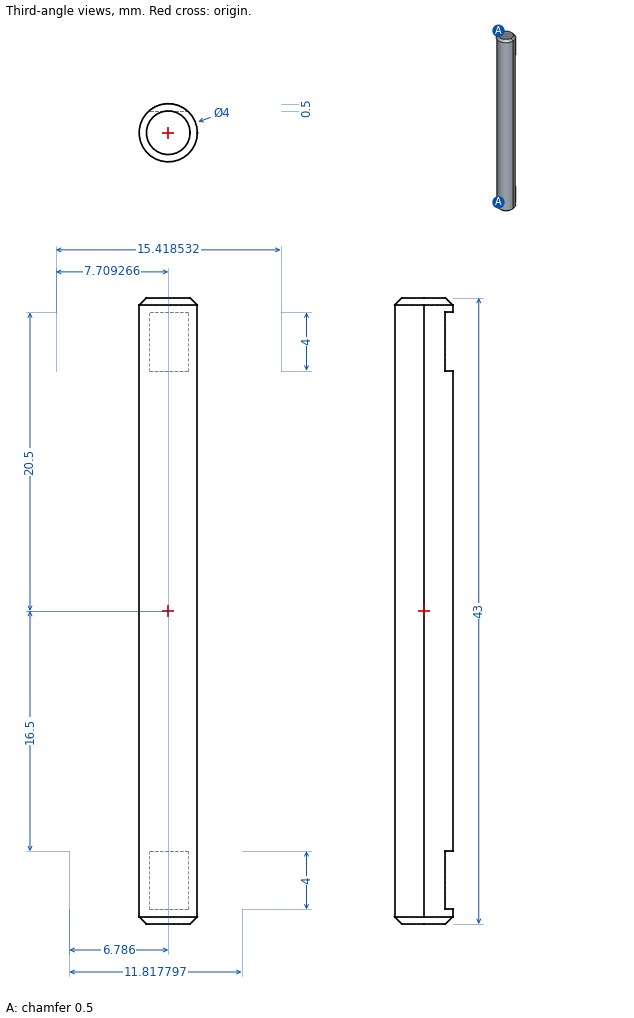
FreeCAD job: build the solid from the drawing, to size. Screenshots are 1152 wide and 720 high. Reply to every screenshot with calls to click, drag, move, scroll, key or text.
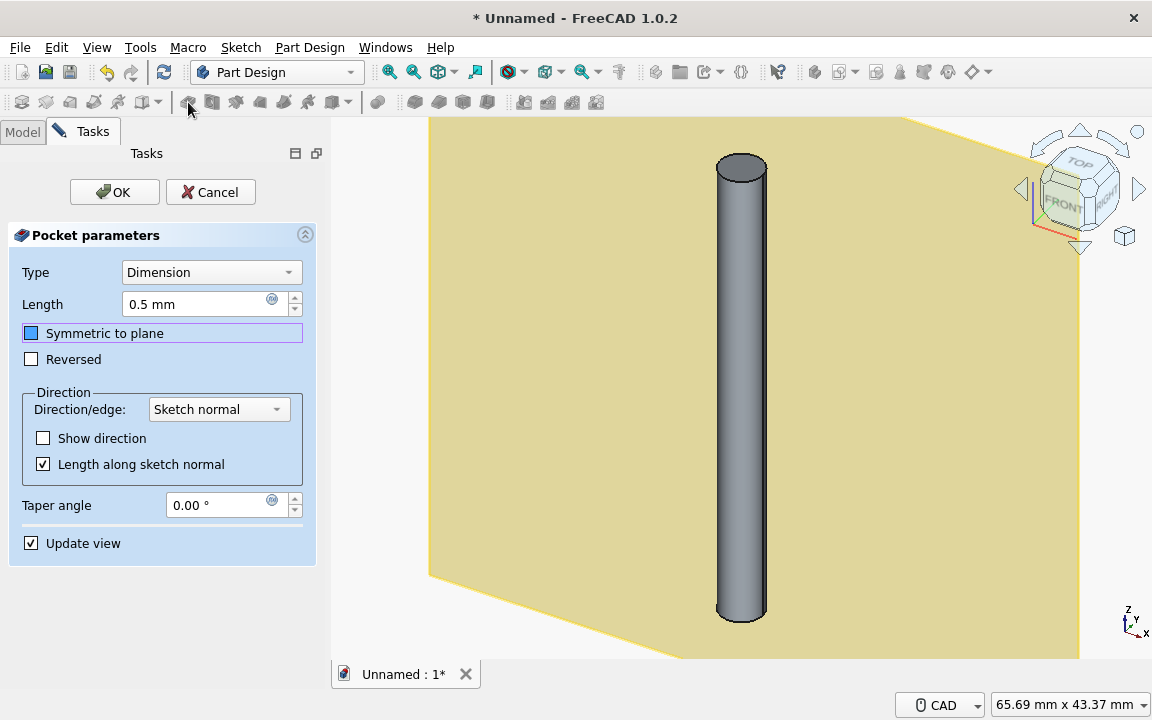
click(30, 359)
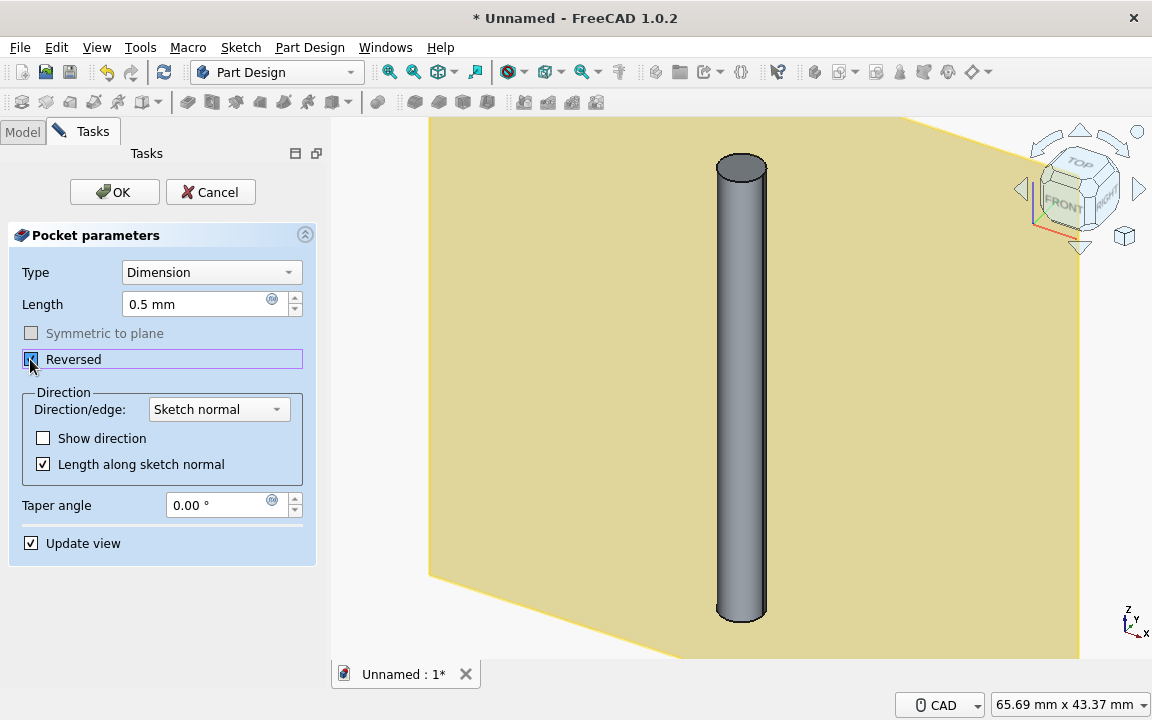
click(115, 192)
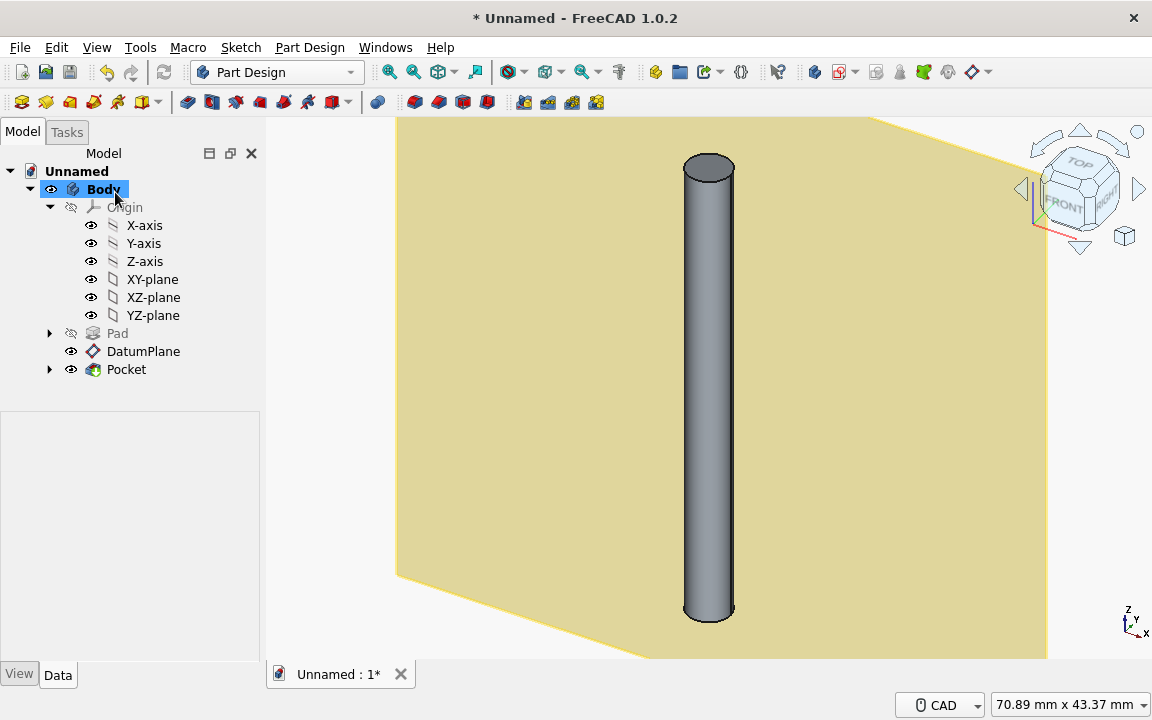
click(116, 351)
key(space)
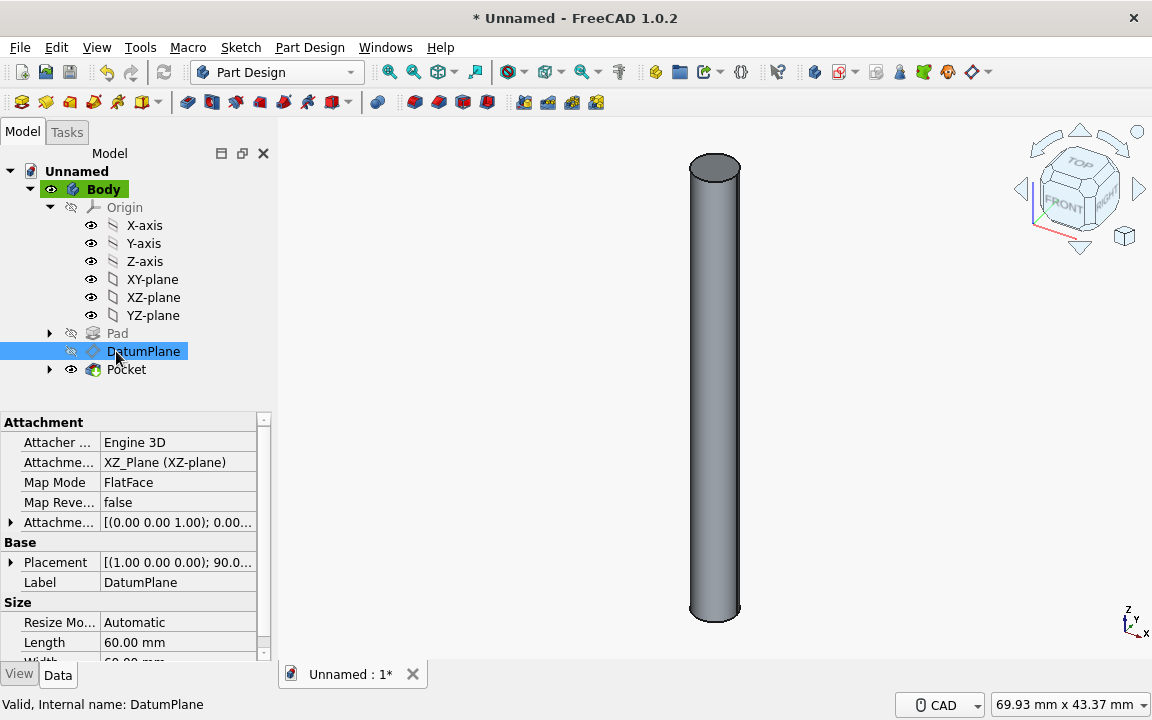
click(696, 617)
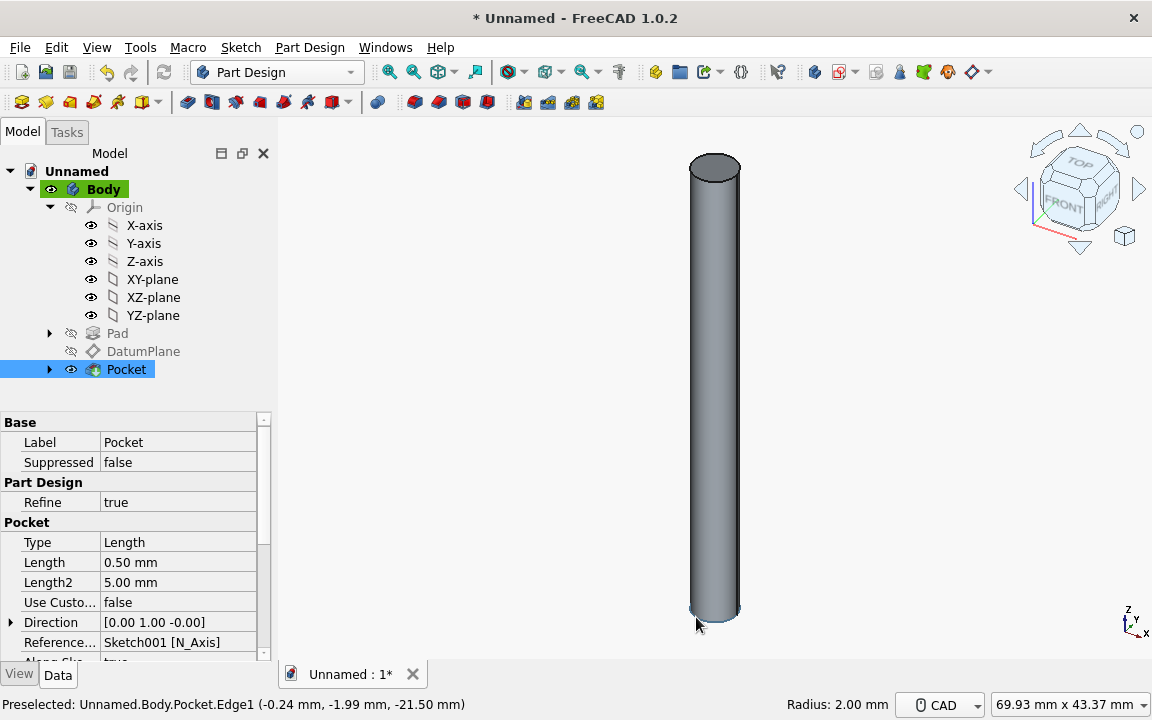
click(693, 160, ctrl)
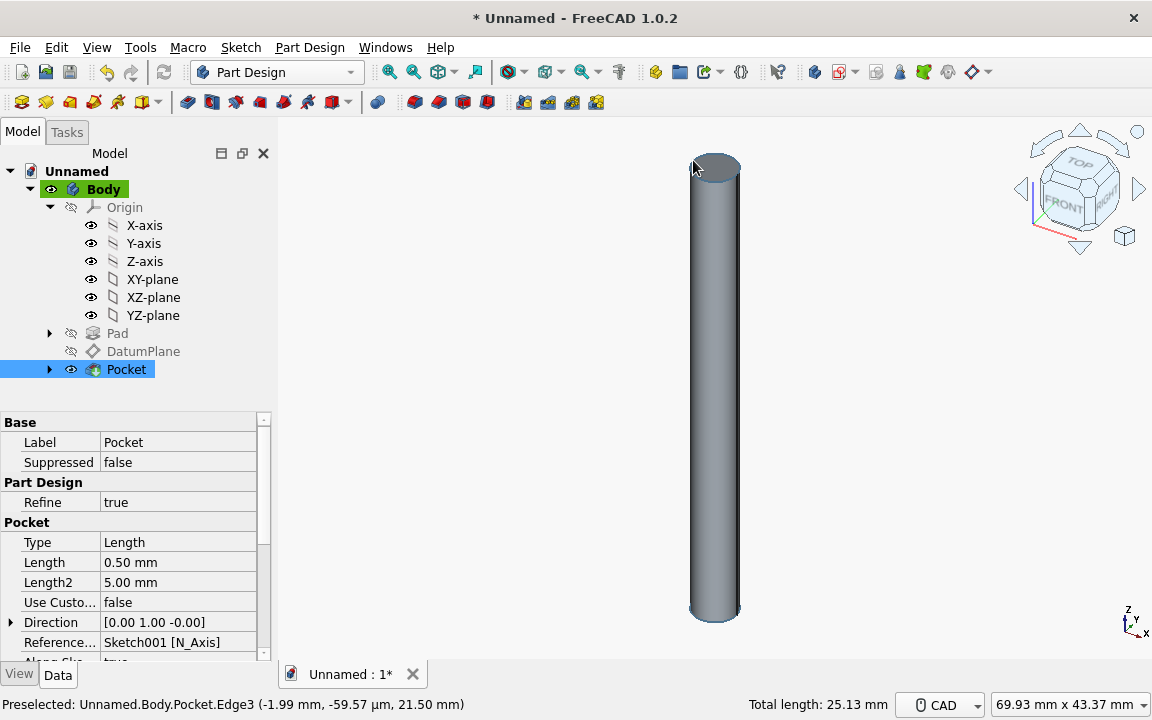
click(440, 102)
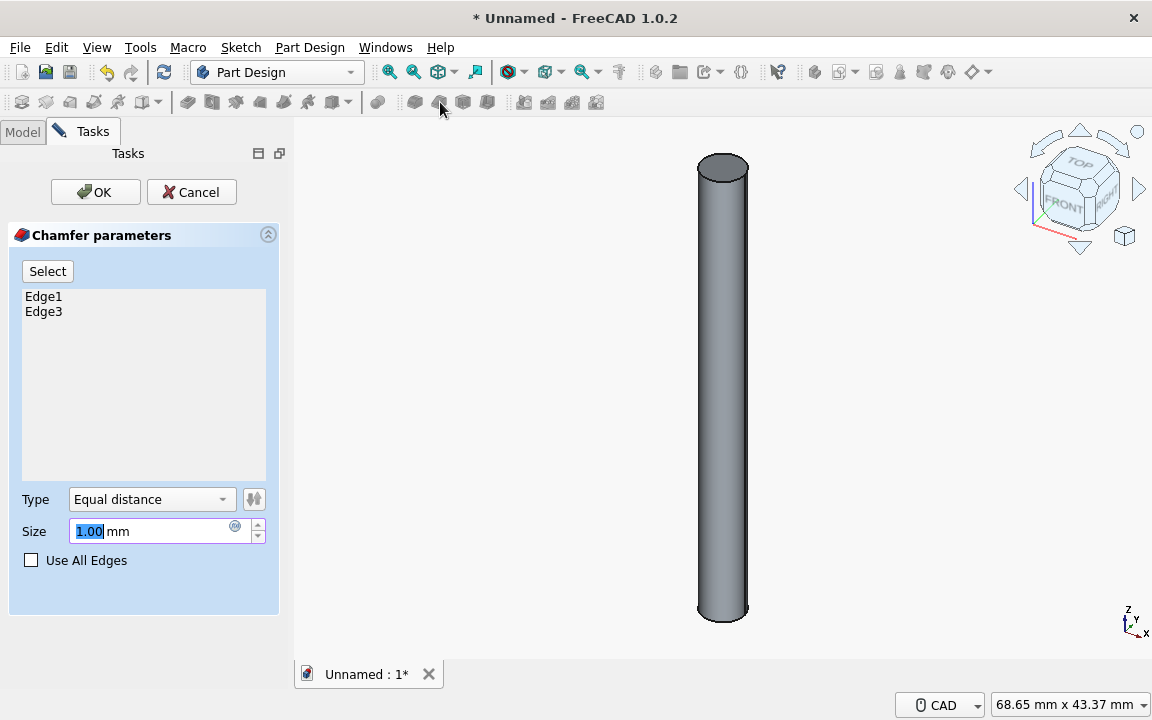
text(0.5)
key(Tab)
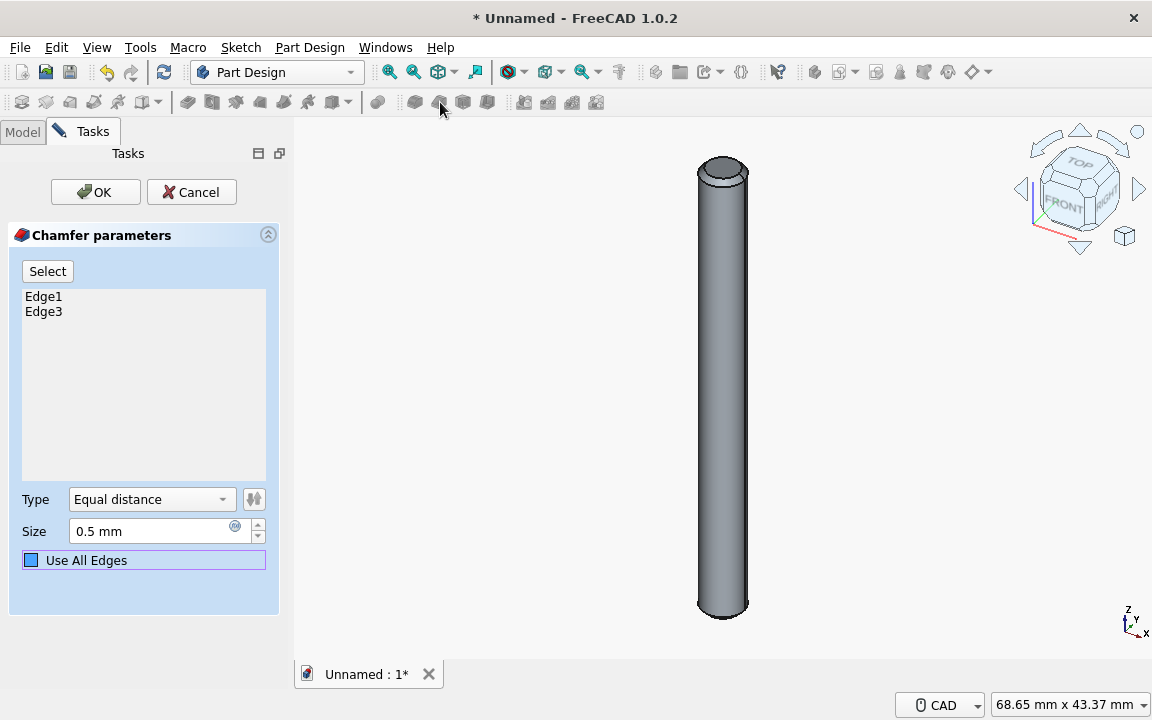
click(96, 192)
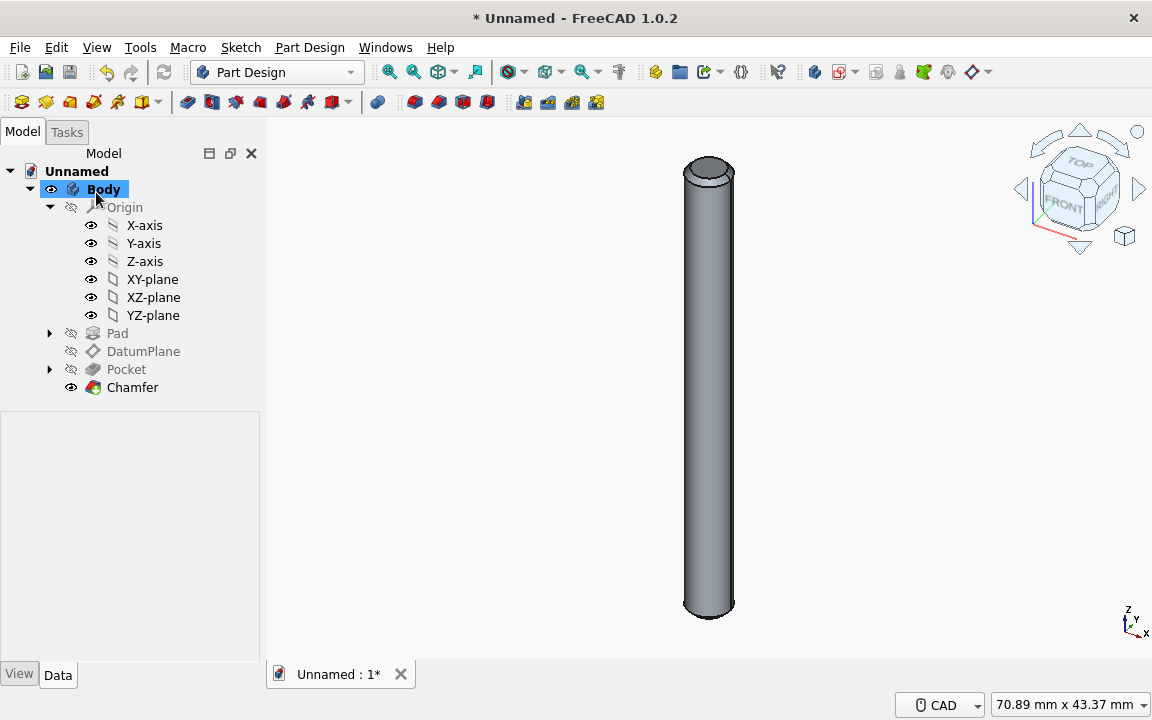
key(0)